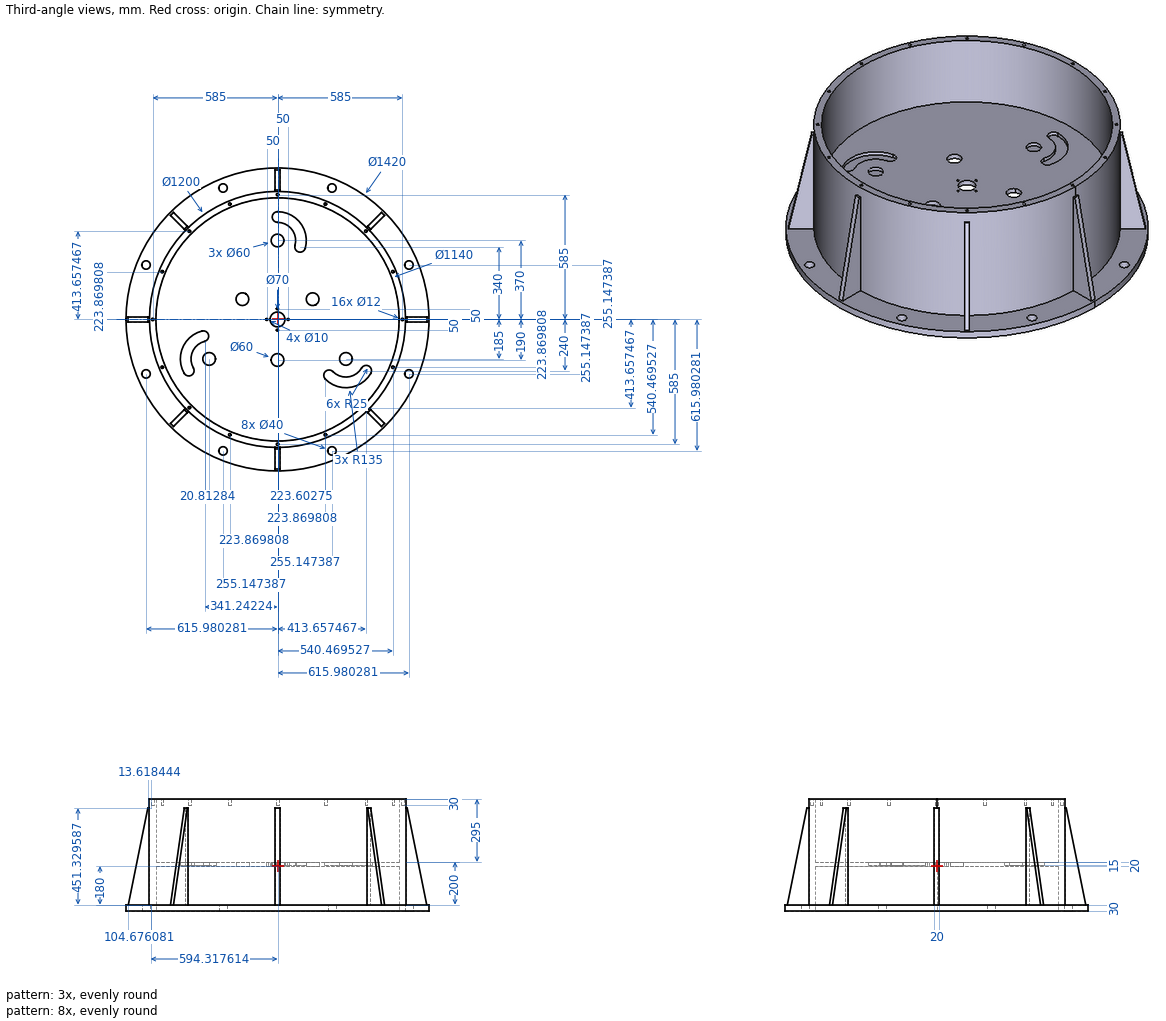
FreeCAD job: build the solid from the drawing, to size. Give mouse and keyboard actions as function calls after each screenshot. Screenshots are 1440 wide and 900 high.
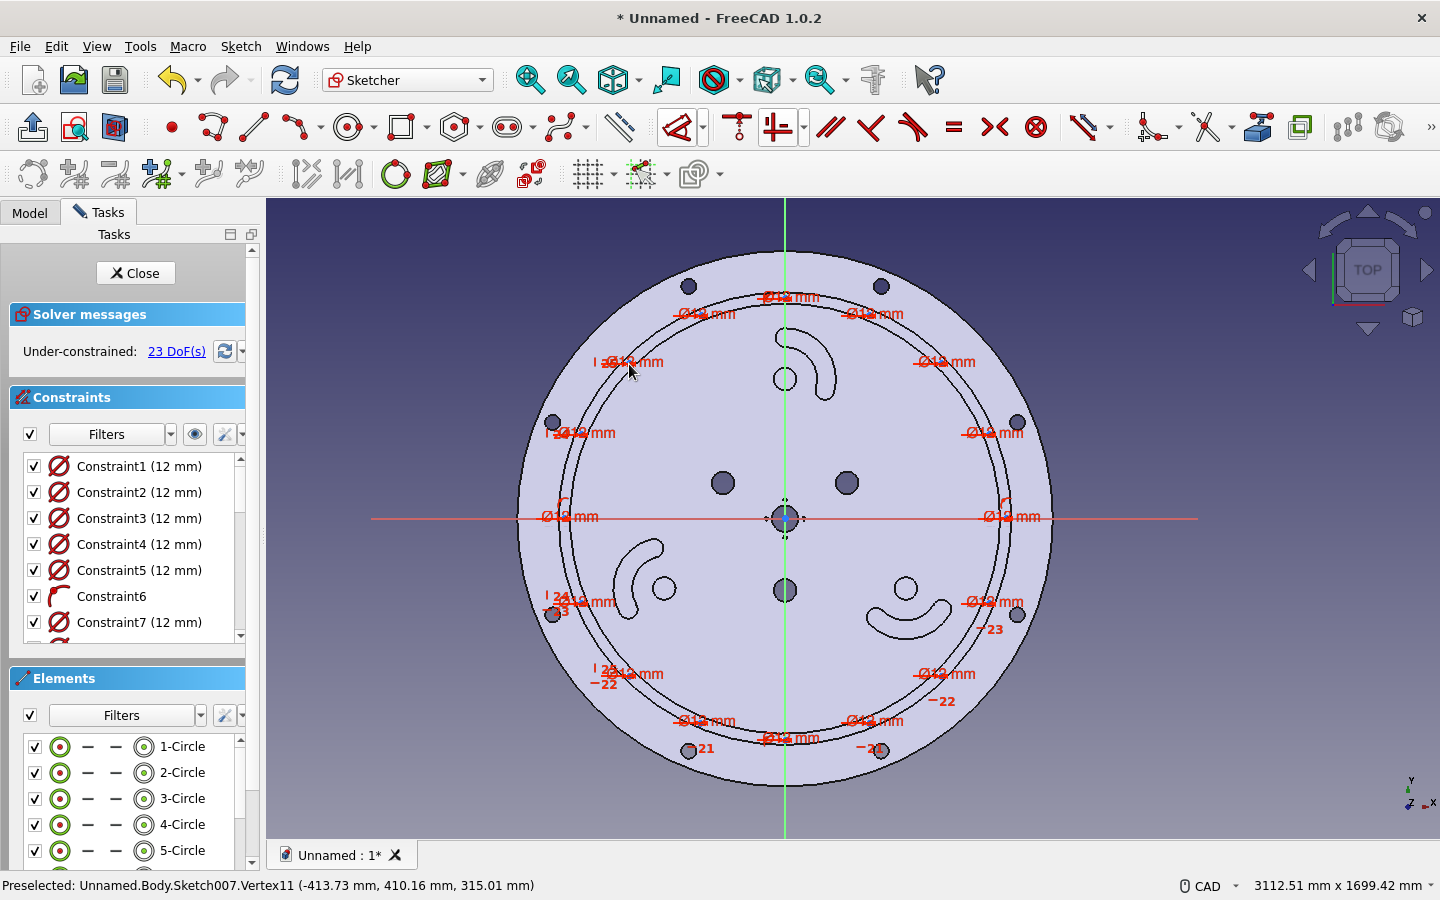
click(701, 316)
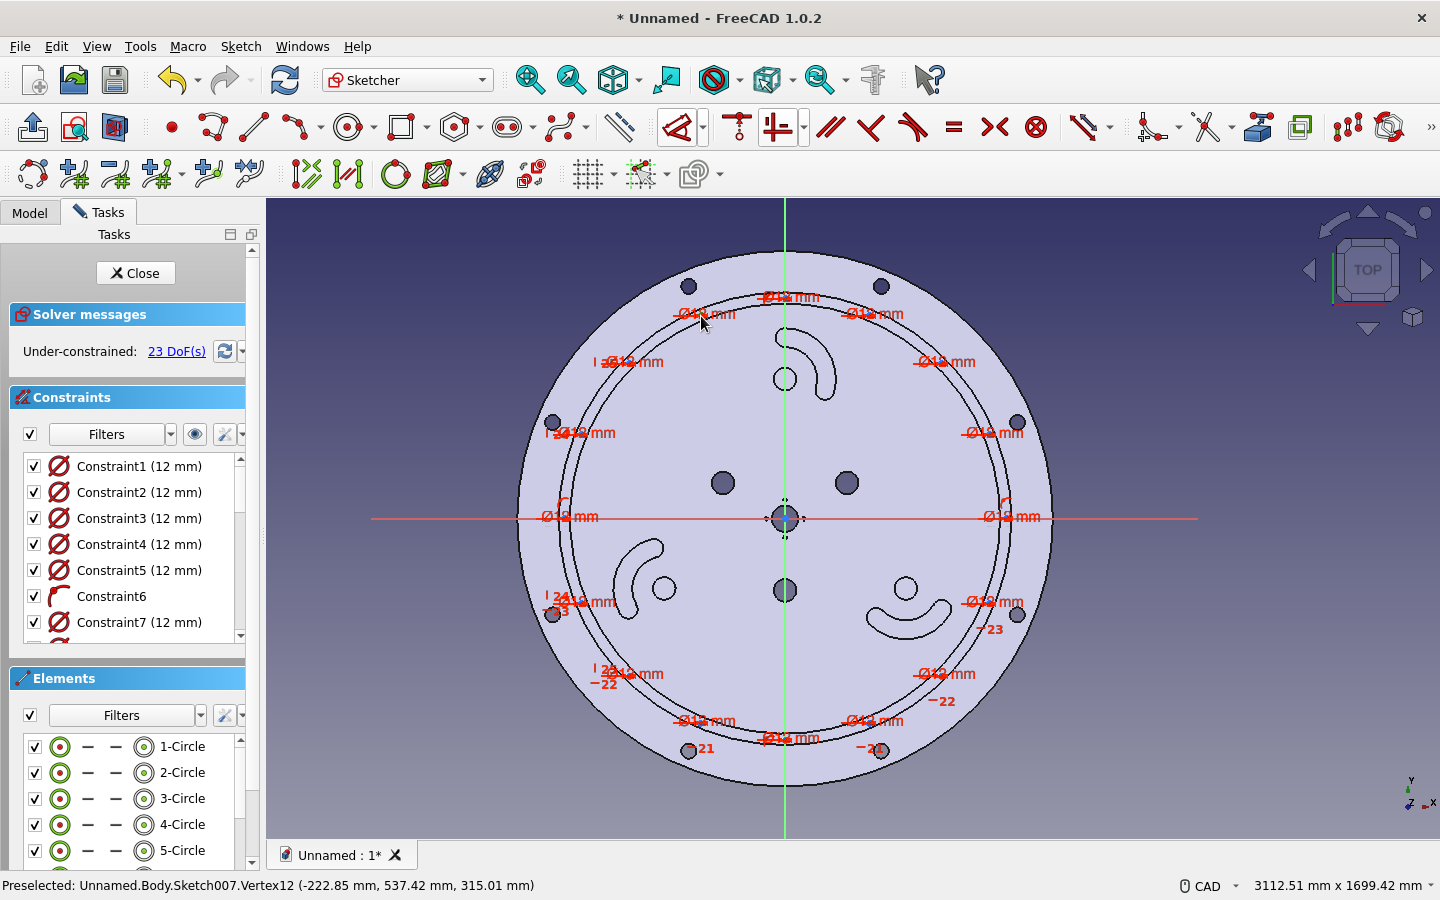
click(869, 316)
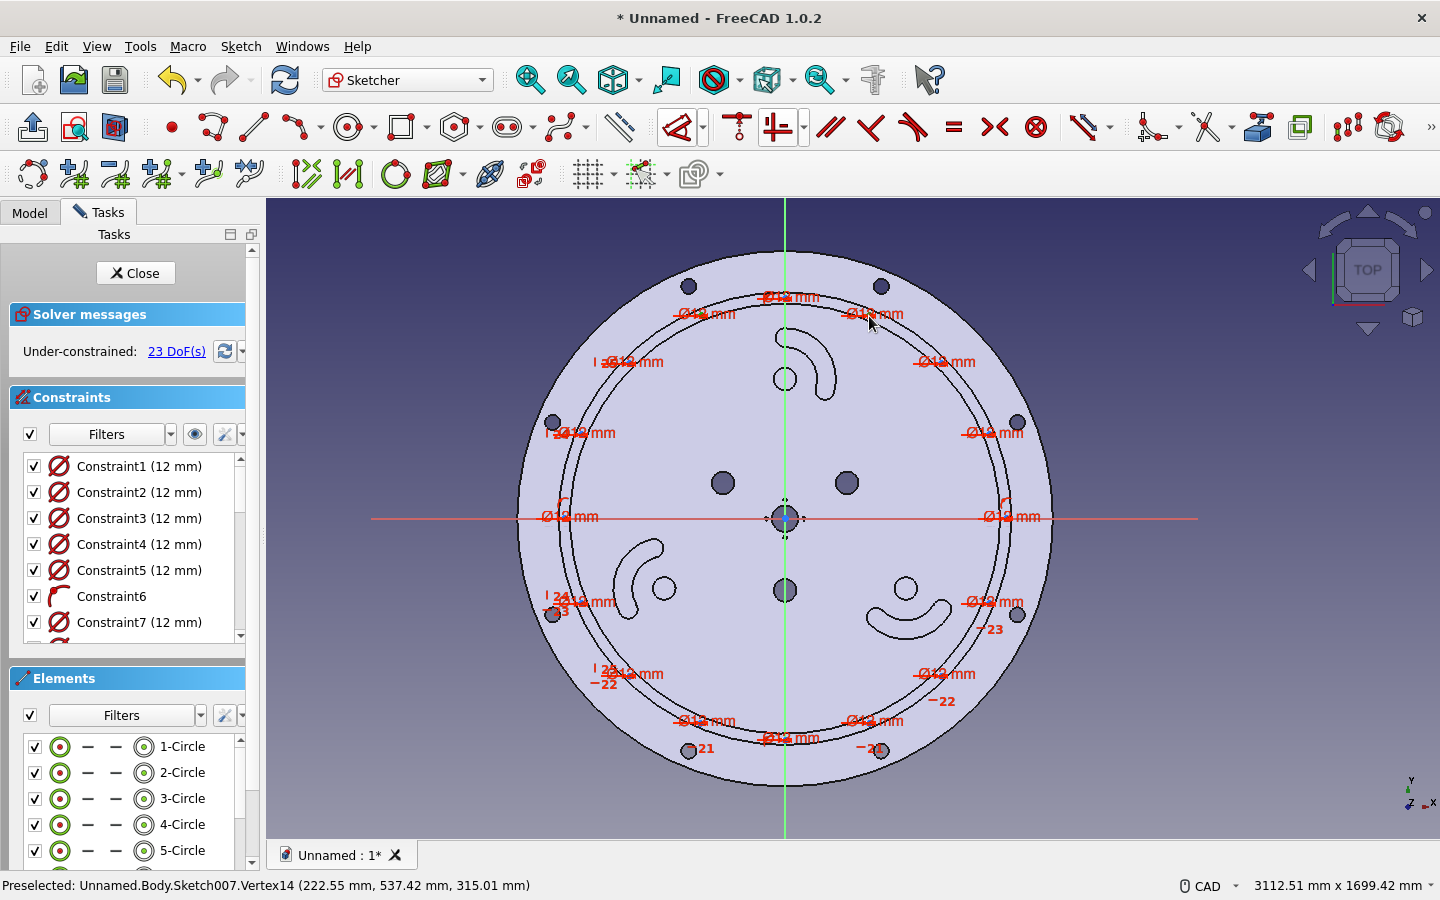
key(h)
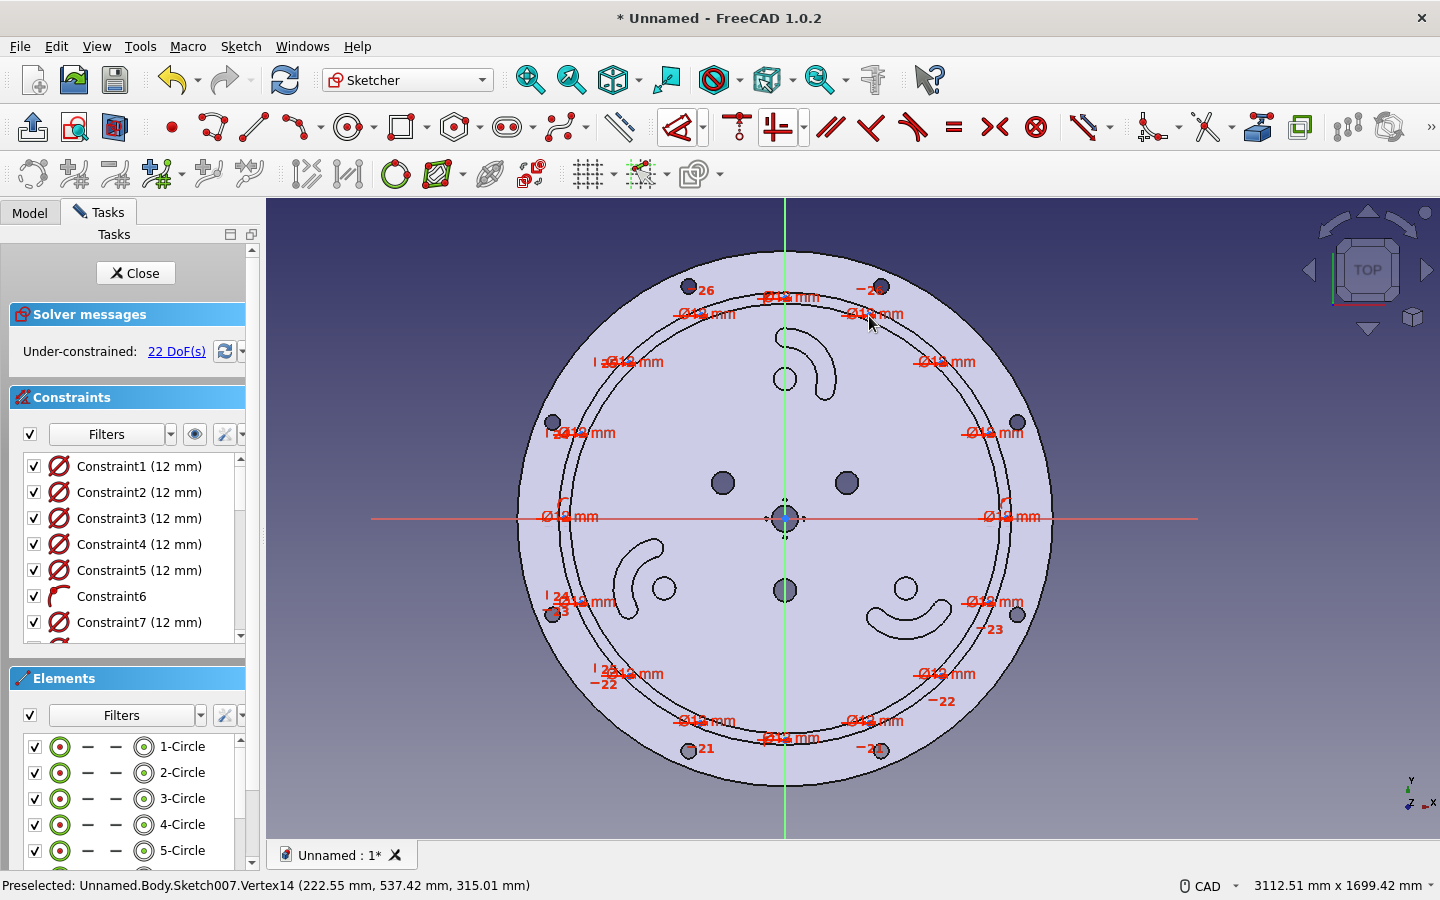
click(941, 676)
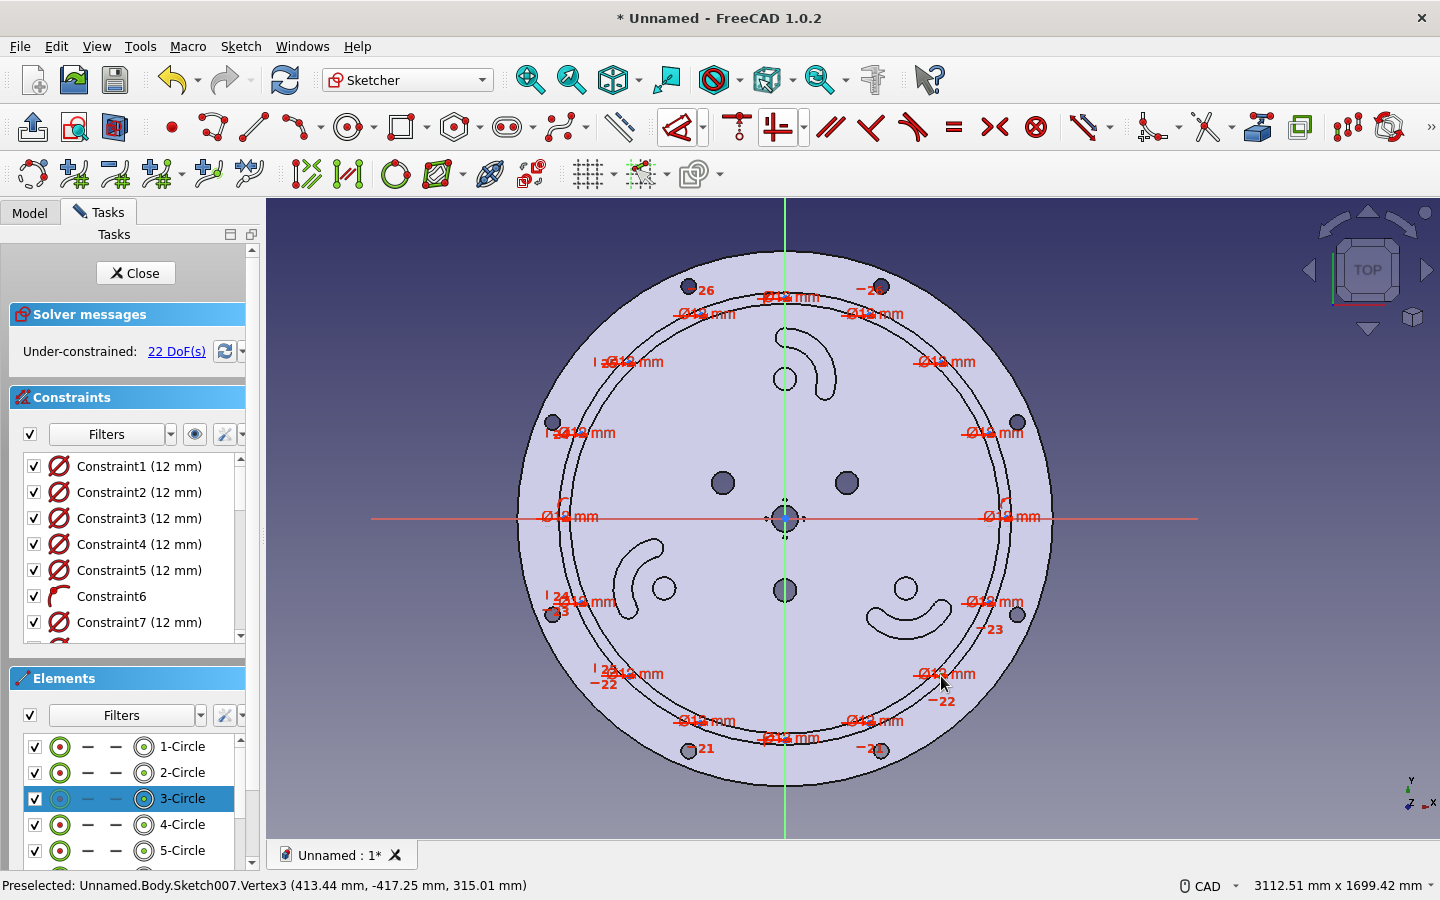
click(941, 364)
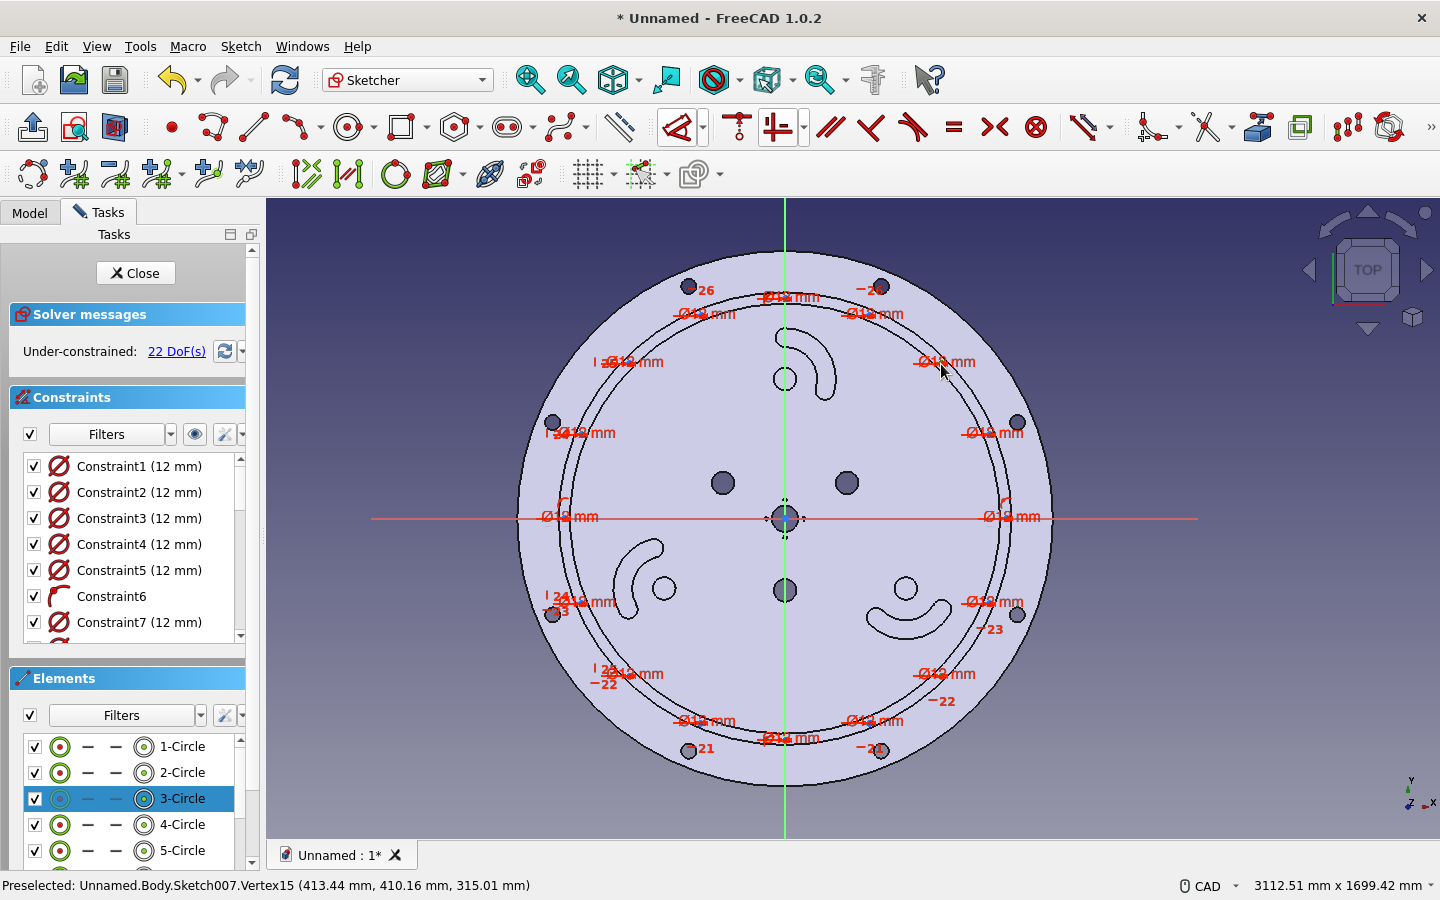
click(804, 128)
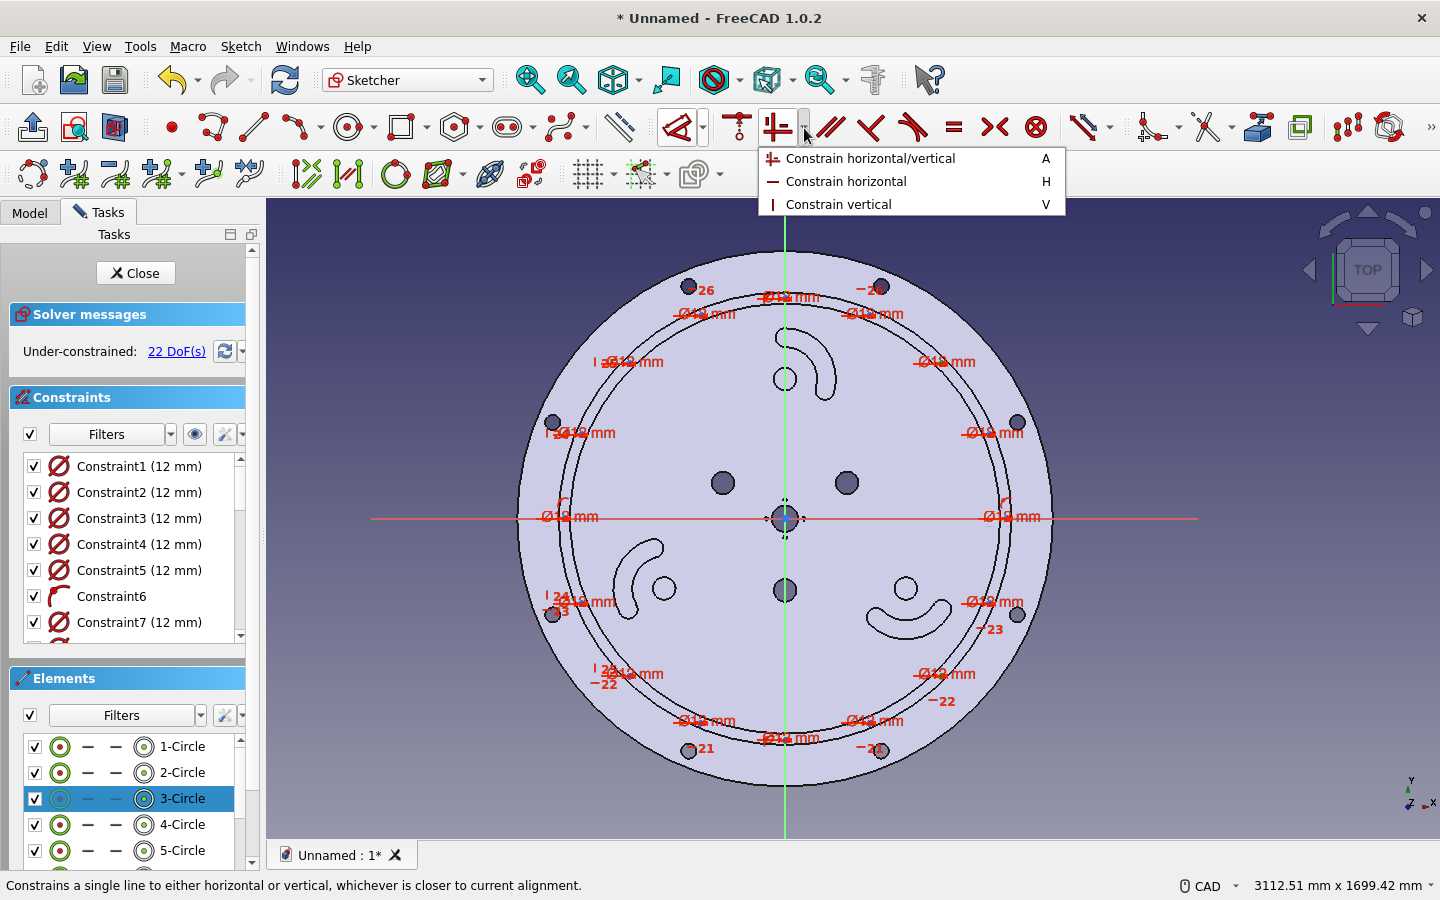
click(912, 204)